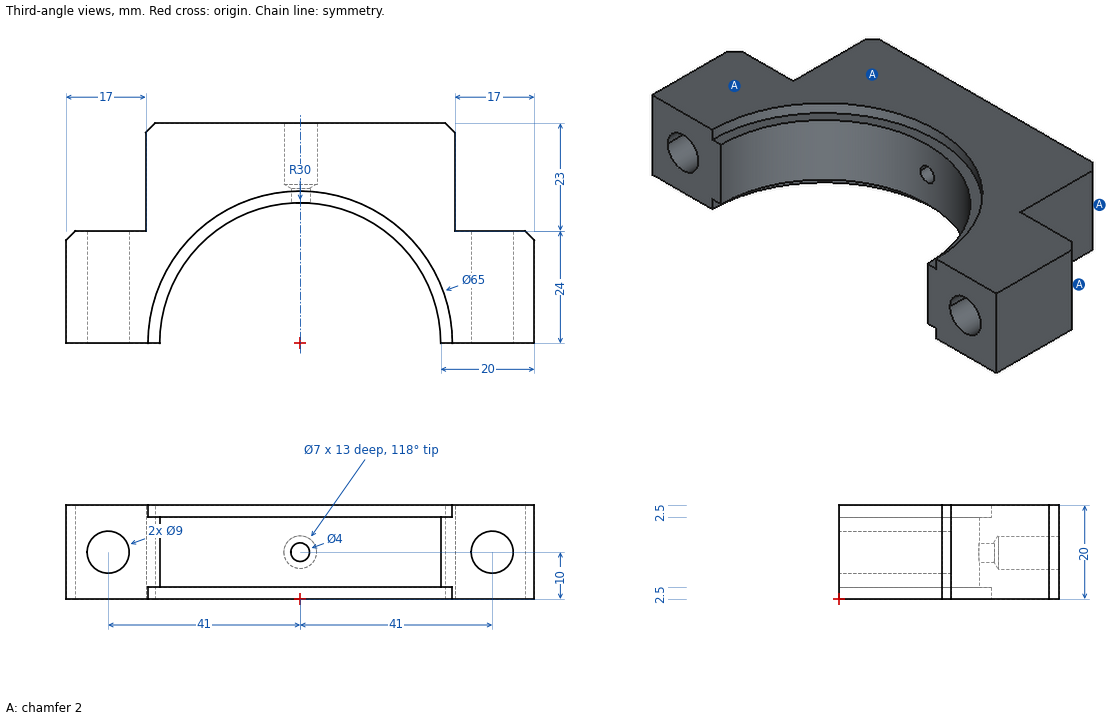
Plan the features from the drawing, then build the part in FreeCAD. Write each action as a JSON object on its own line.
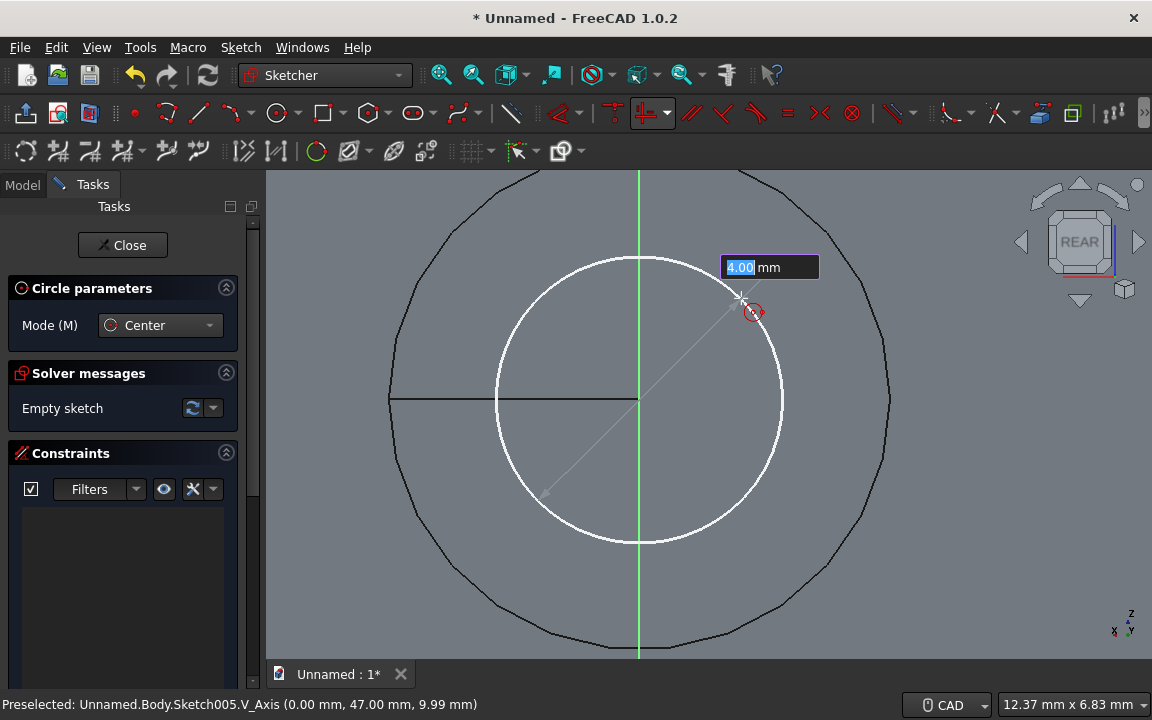
{"action": "type", "text": "4"}
{"action": "key", "text": "Return"}
{"action": "key", "text": "Escape"}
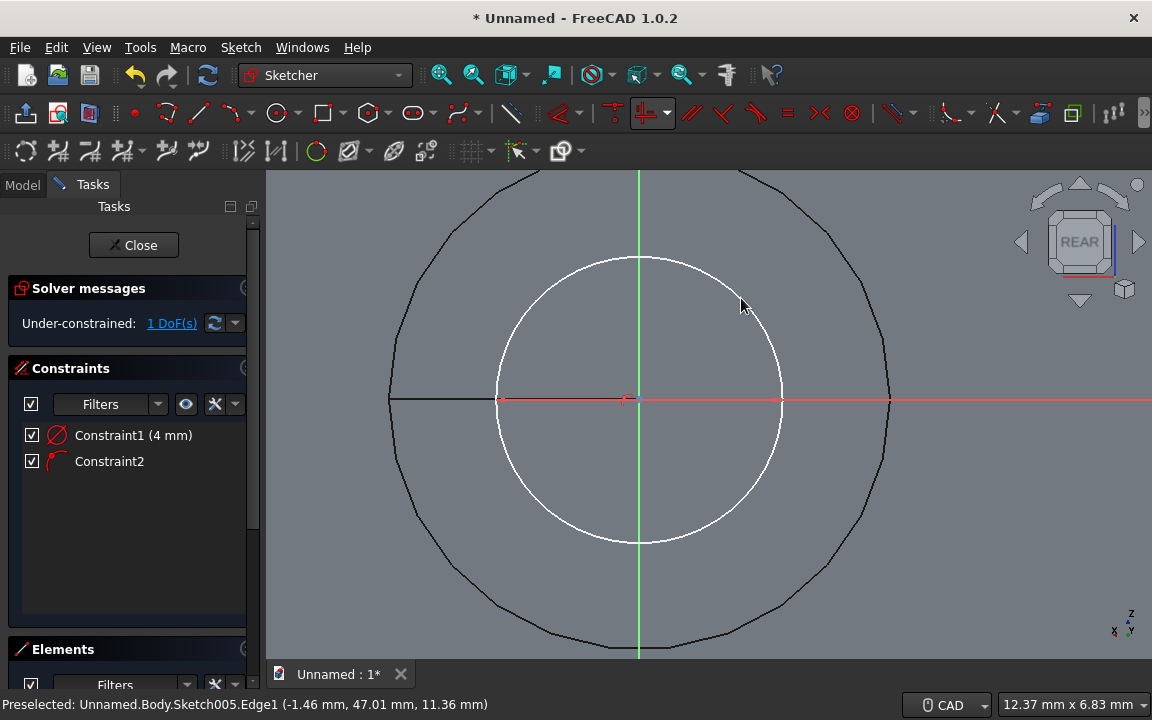
{"action": "left_click", "coordinate": [558, 114]}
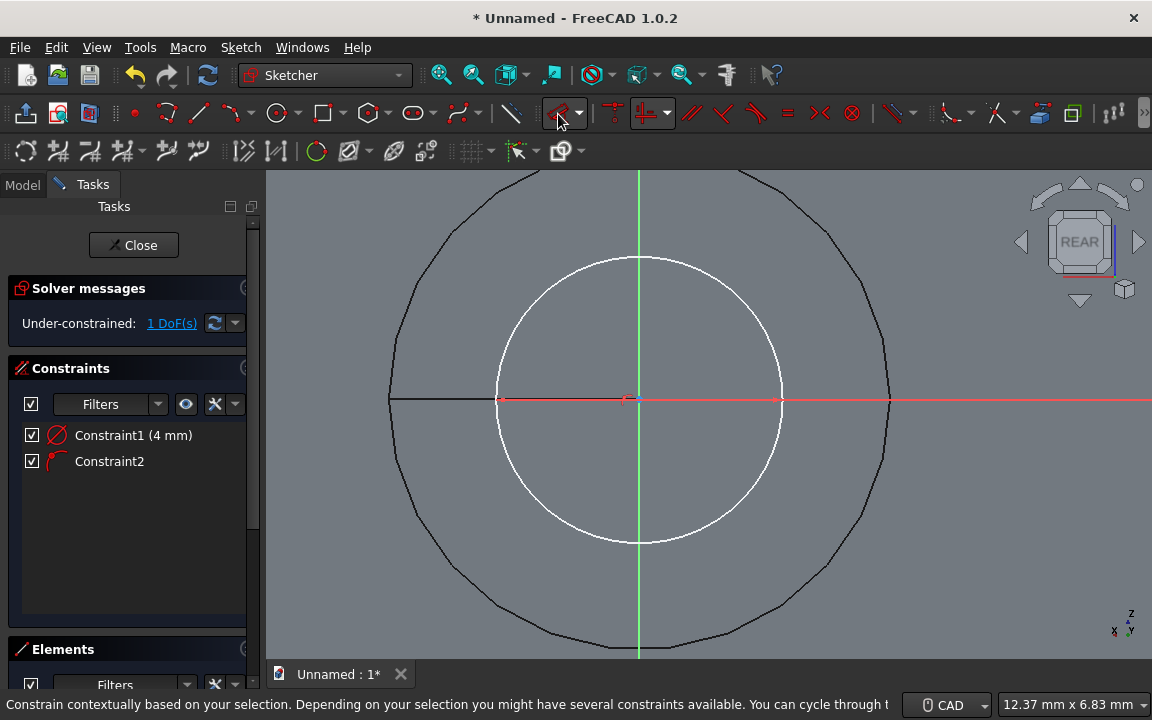
{"action": "left_click", "coordinate": [639, 400]}
{"action": "left_click", "coordinate": [673, 515]}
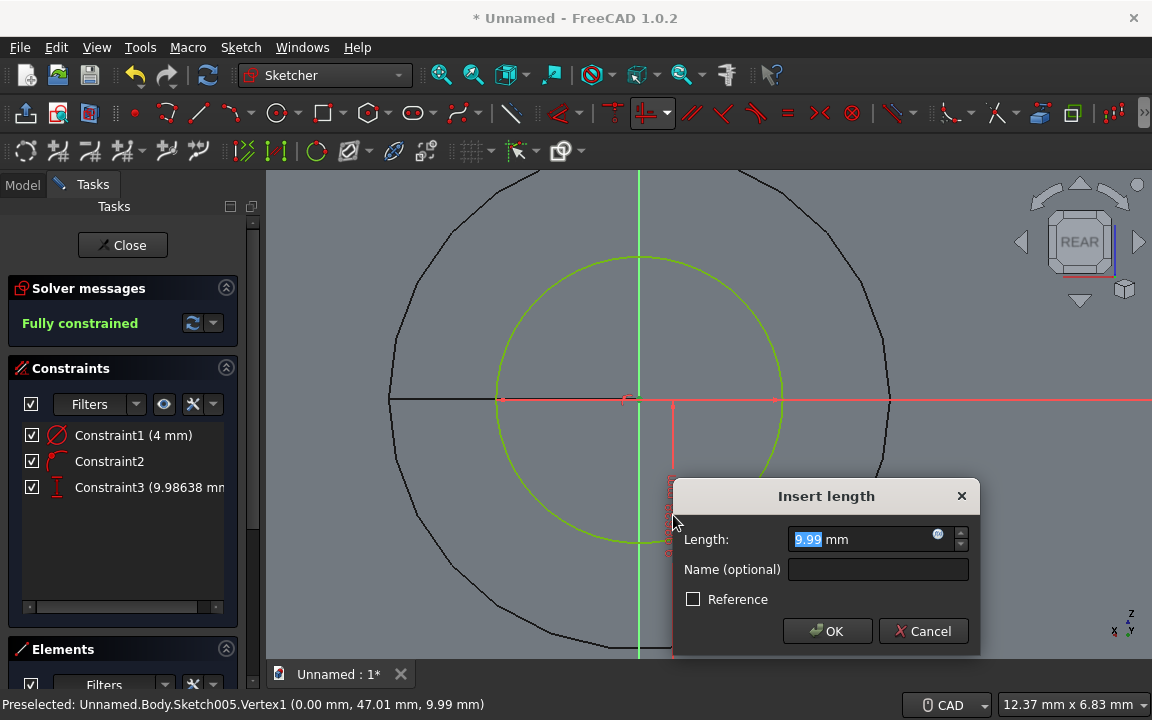
{"action": "type", "text": "10"}
{"action": "key", "text": "Return"}
{"action": "key", "text": "Escape"}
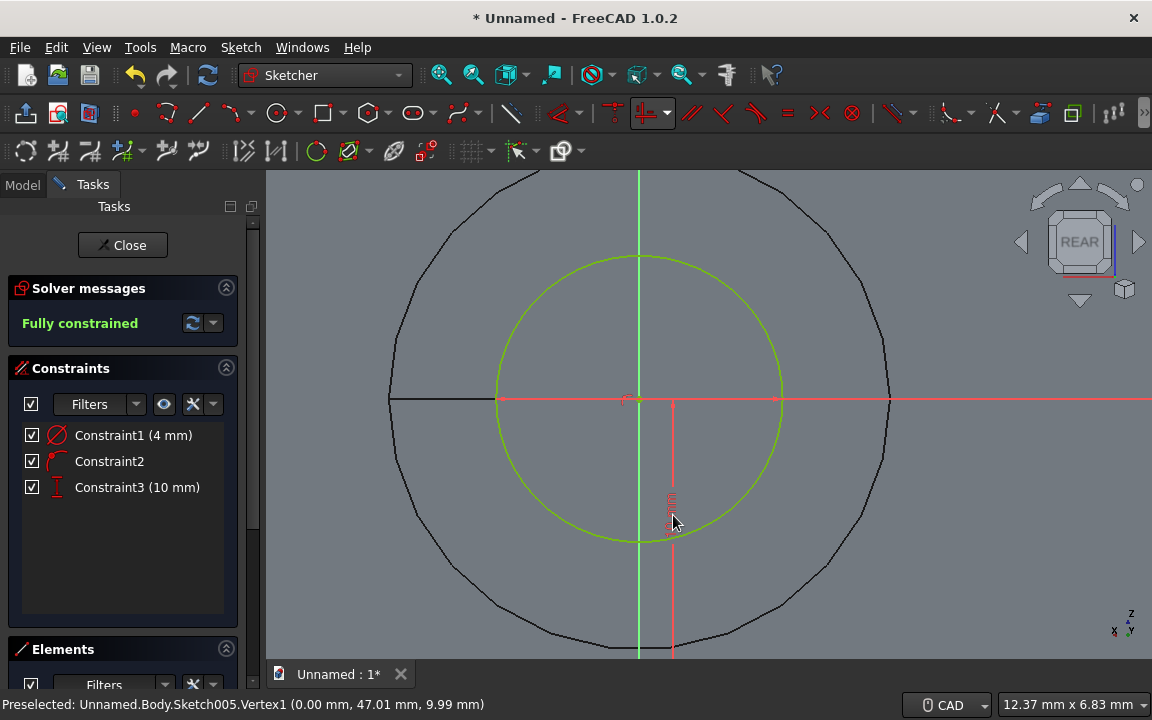
{"action": "left_click", "coordinate": [123, 245]}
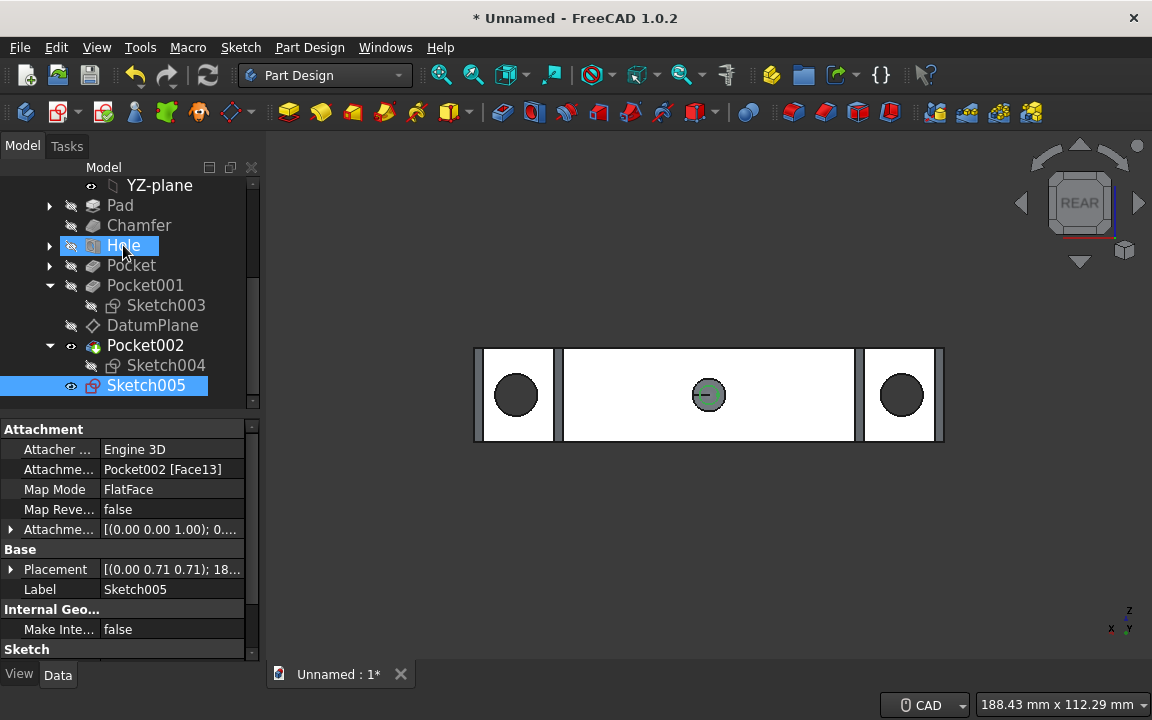
{"action": "left_click", "coordinate": [504, 112]}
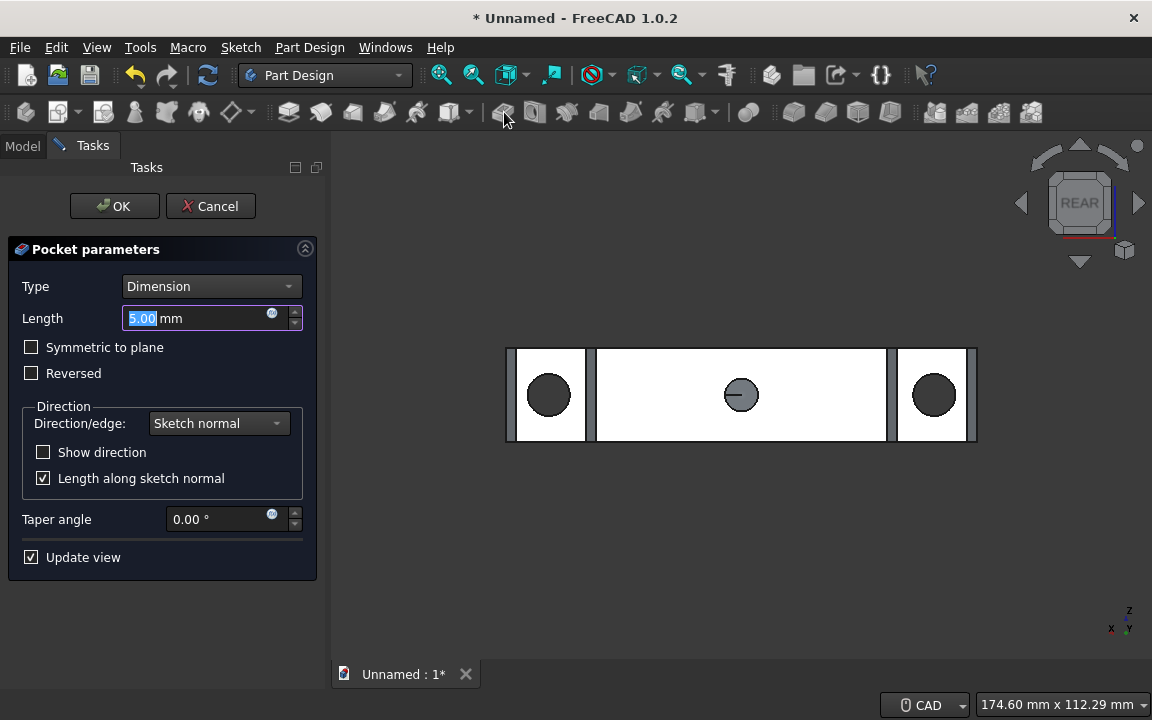
{"action": "left_click", "coordinate": [212, 286]}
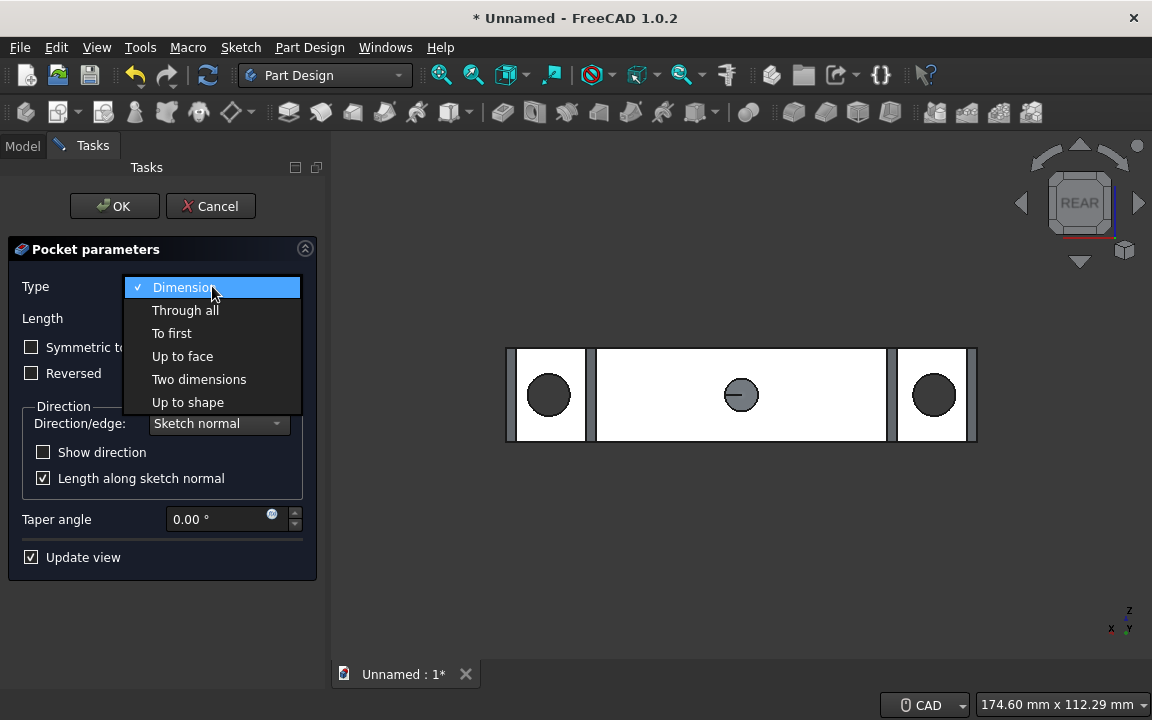
{"action": "left_click", "coordinate": [212, 310]}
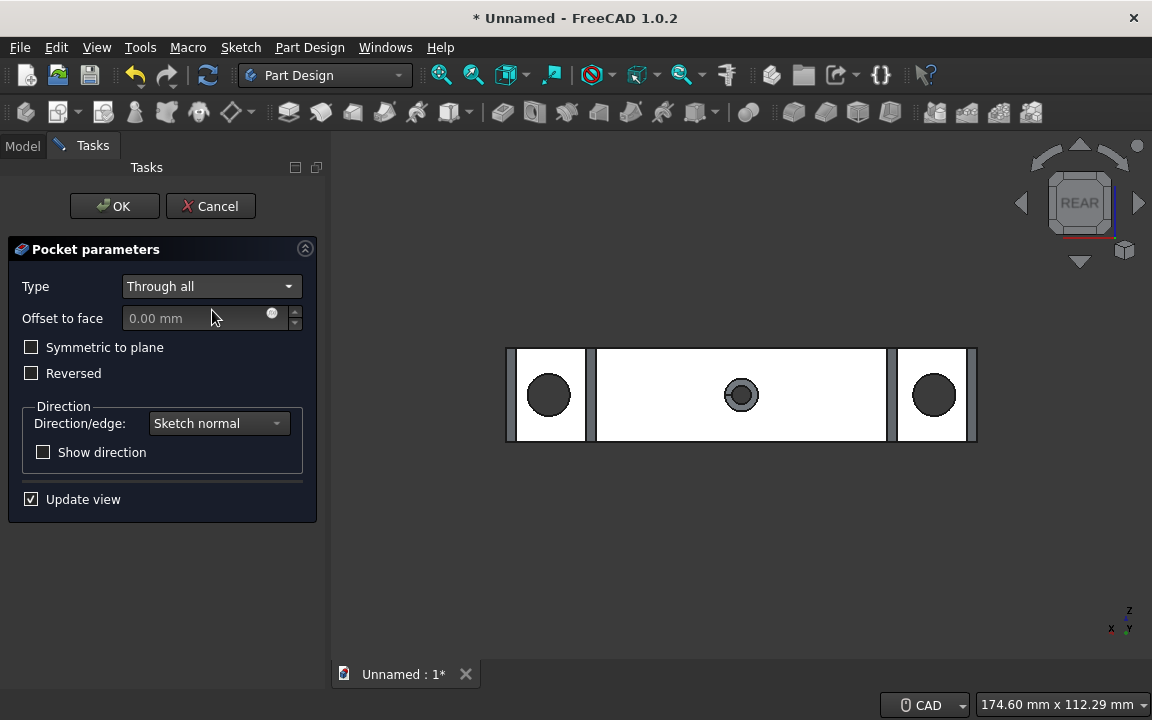
{"action": "left_click", "coordinate": [115, 206]}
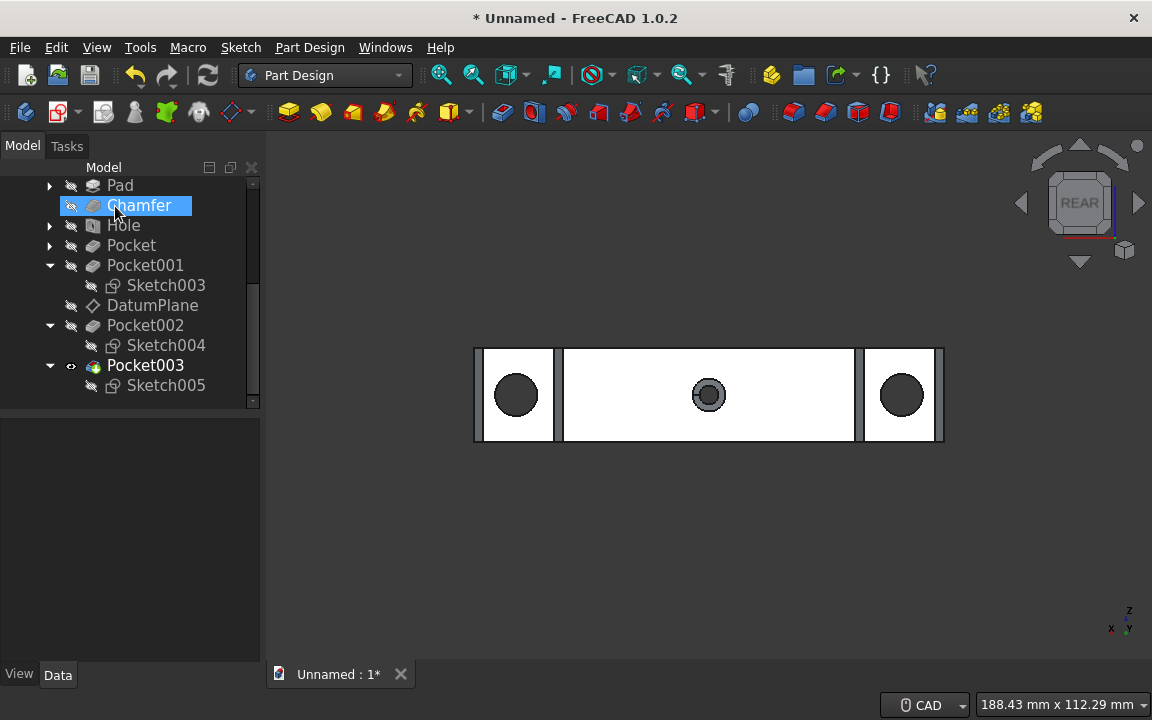
{"action": "key", "text": "0"}